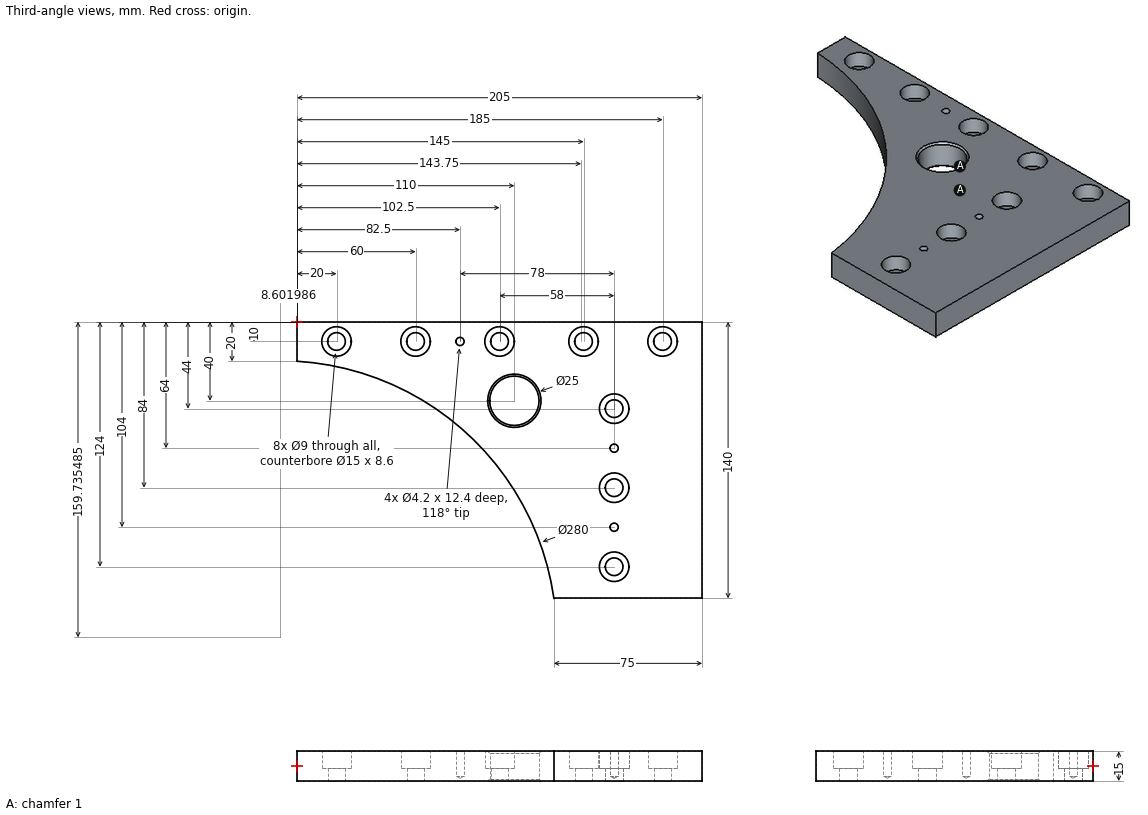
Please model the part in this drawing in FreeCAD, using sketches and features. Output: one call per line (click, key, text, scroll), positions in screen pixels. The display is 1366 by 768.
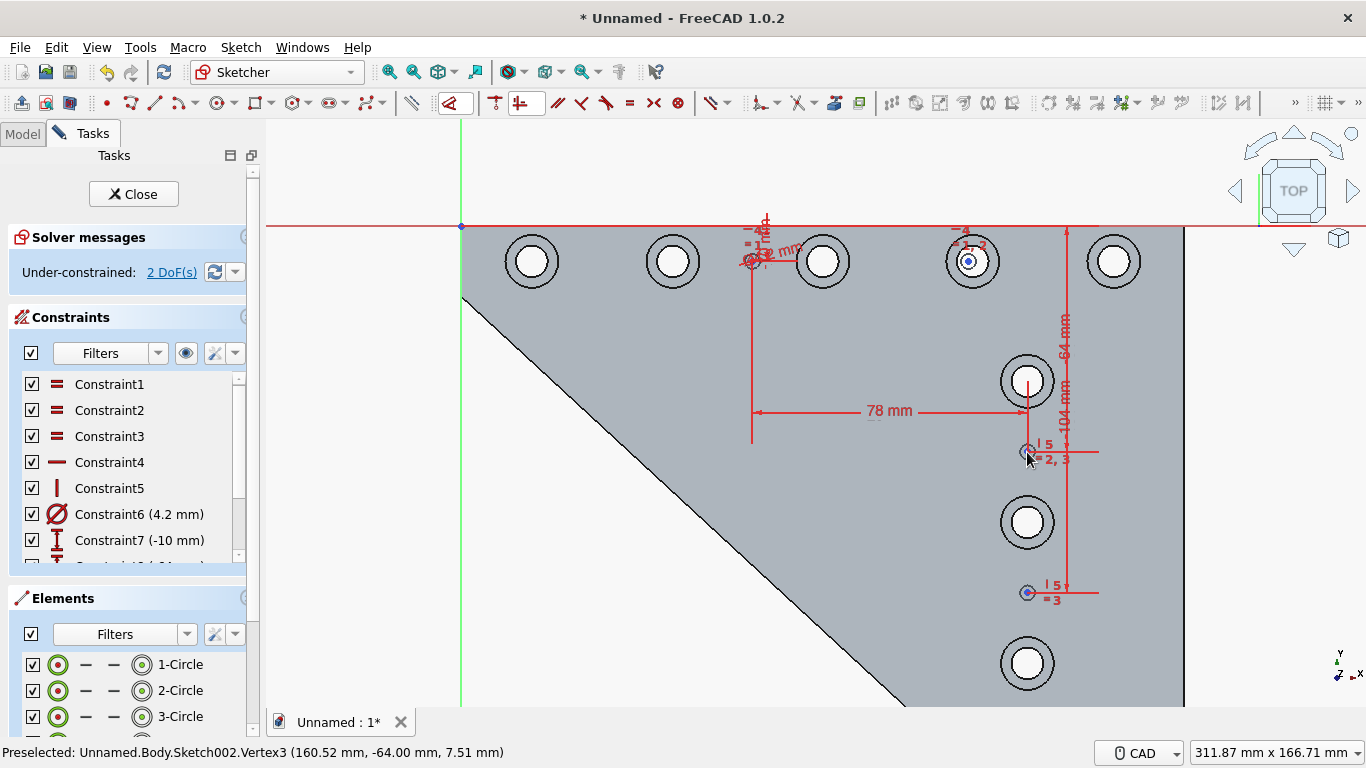
click(752, 261)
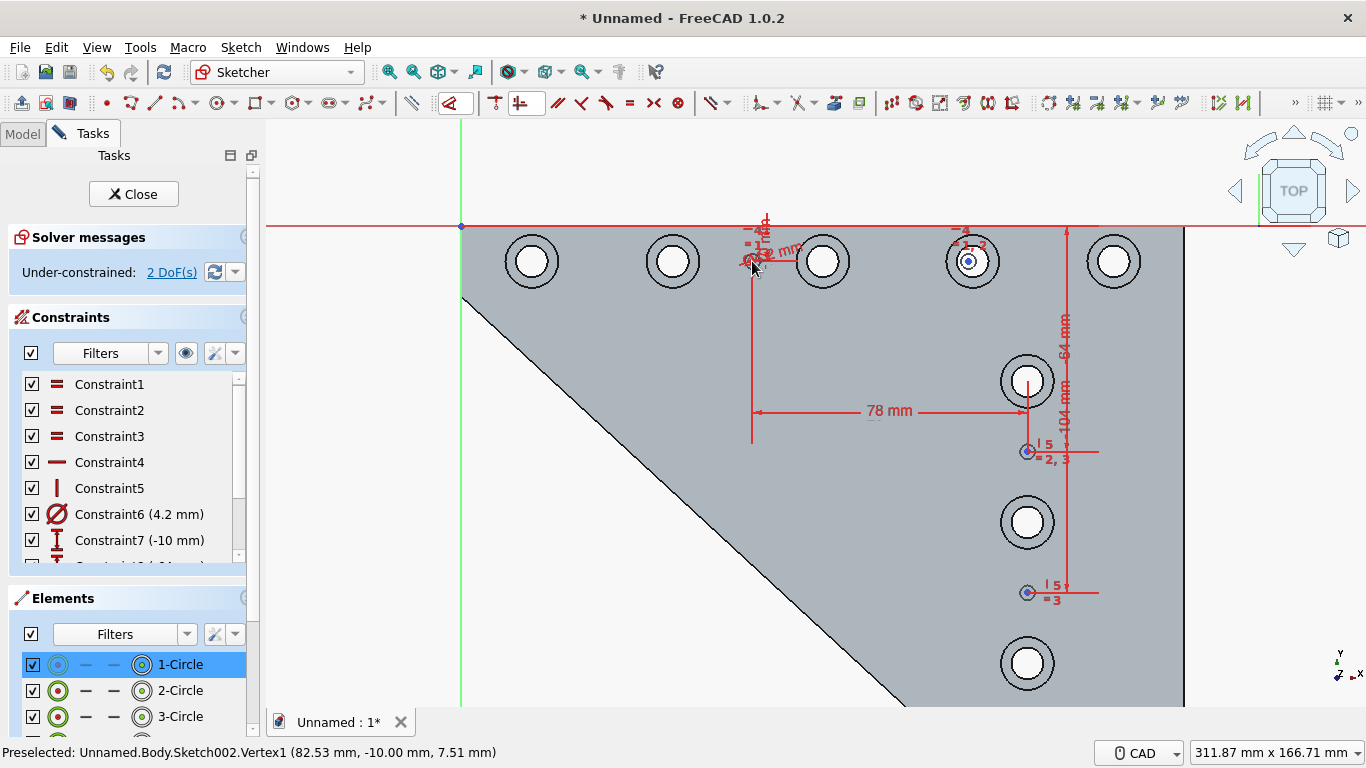
click(468, 104)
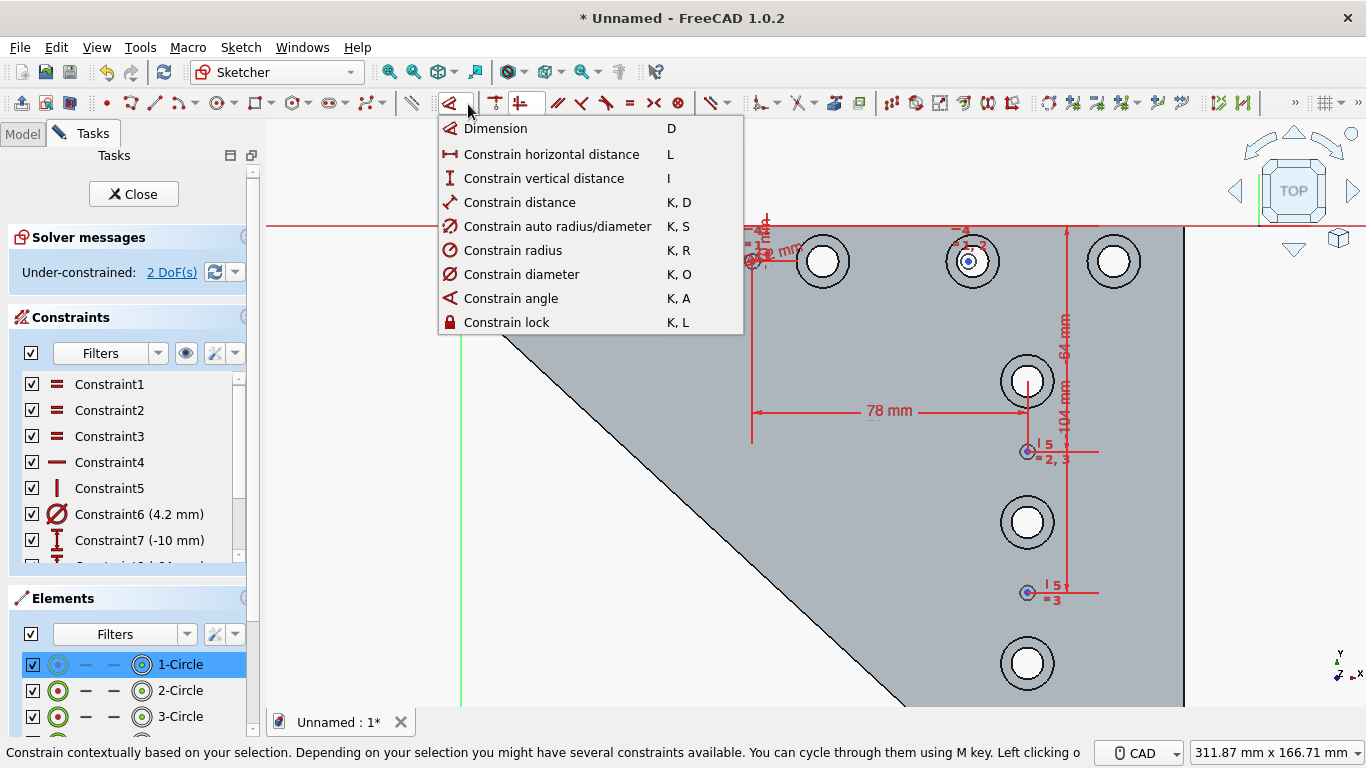
click(591, 154)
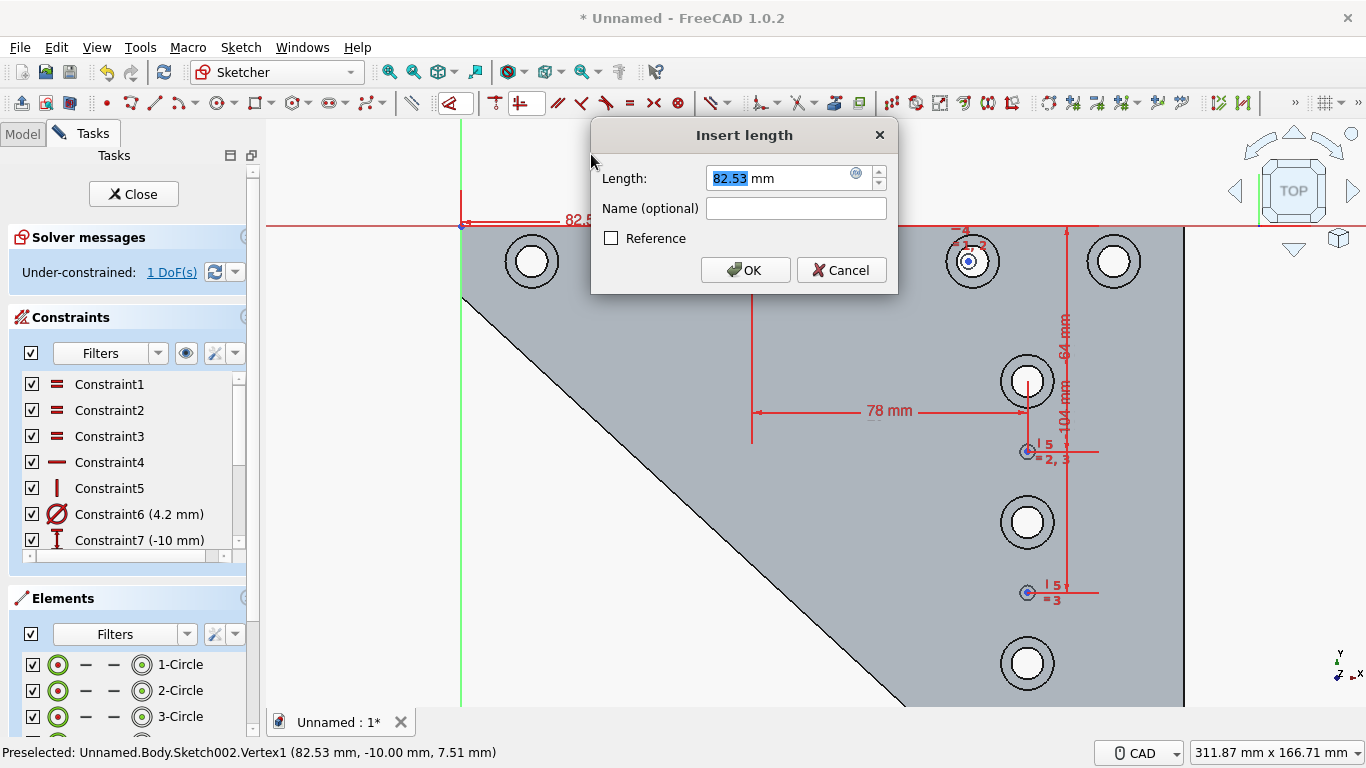
text(82.5)
key(Return)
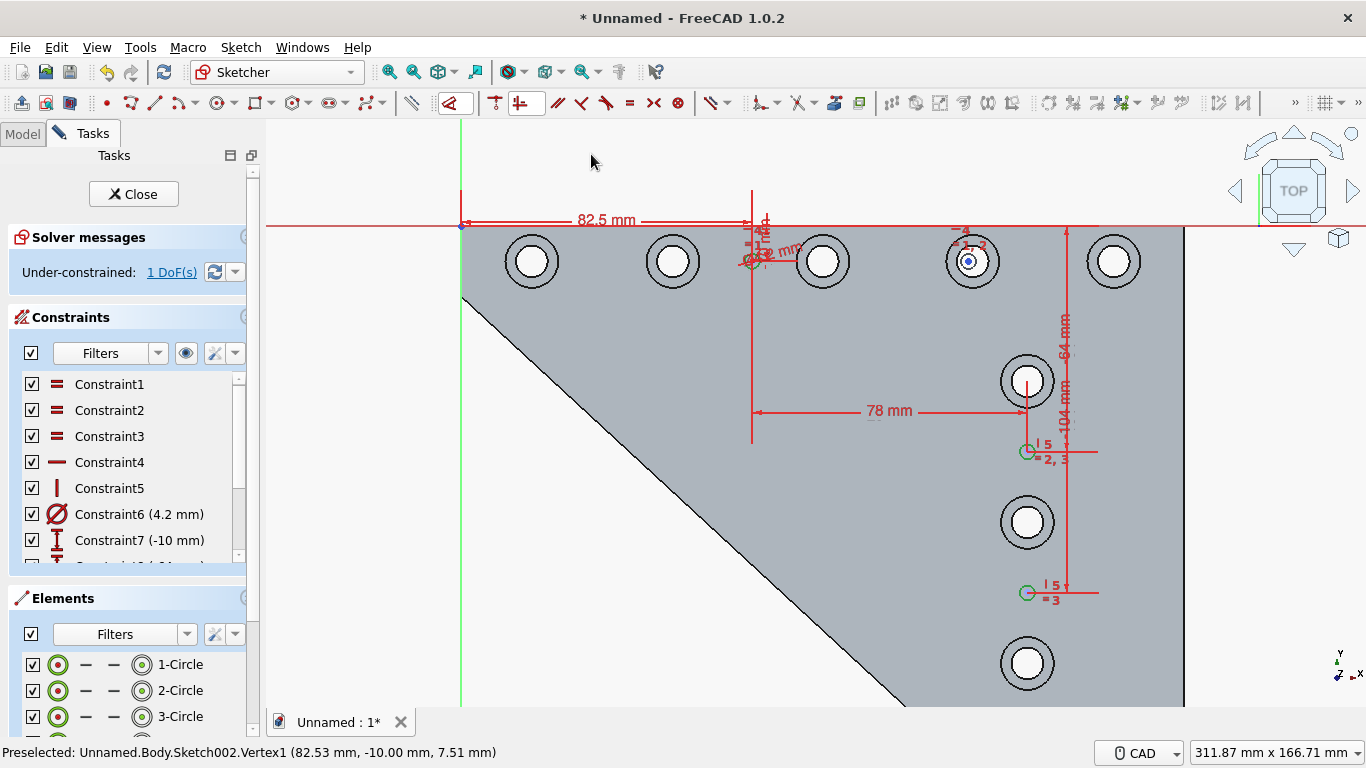
click(968, 261)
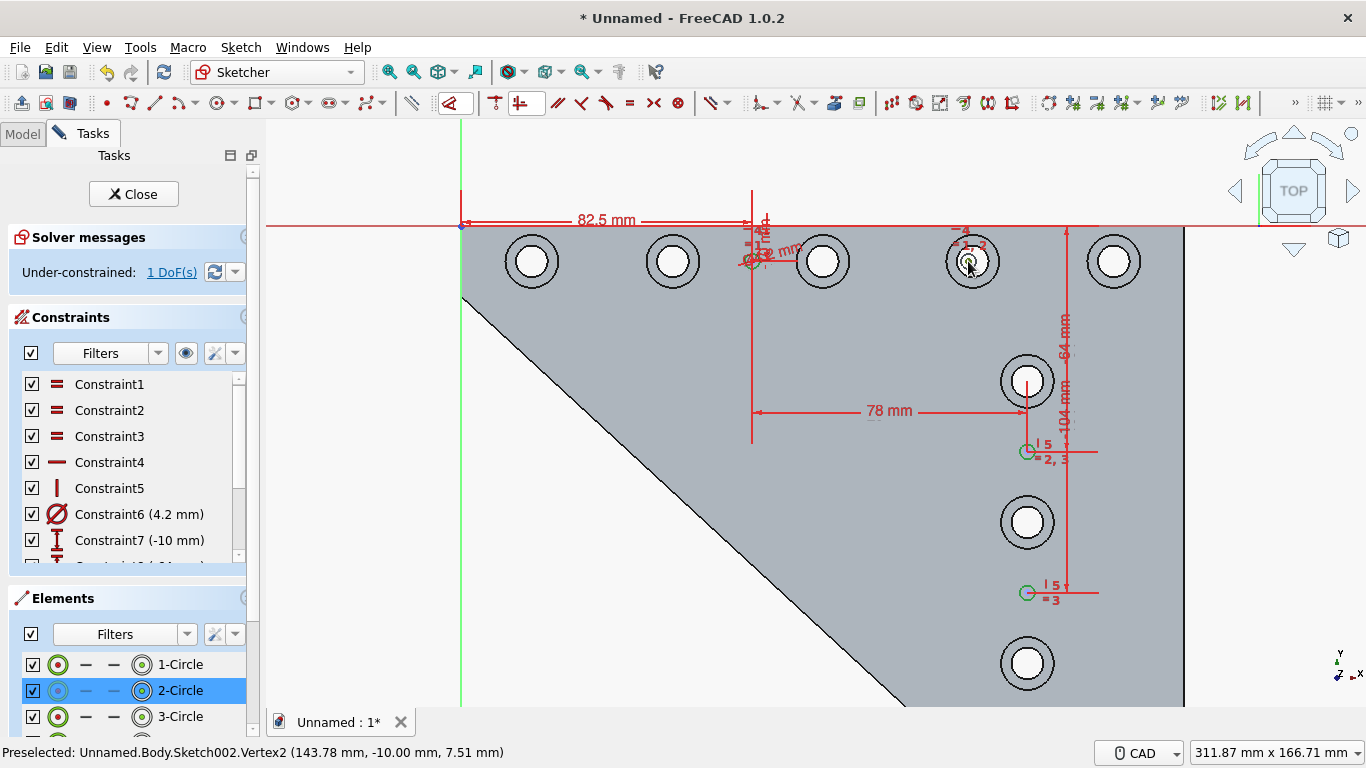
click(468, 104)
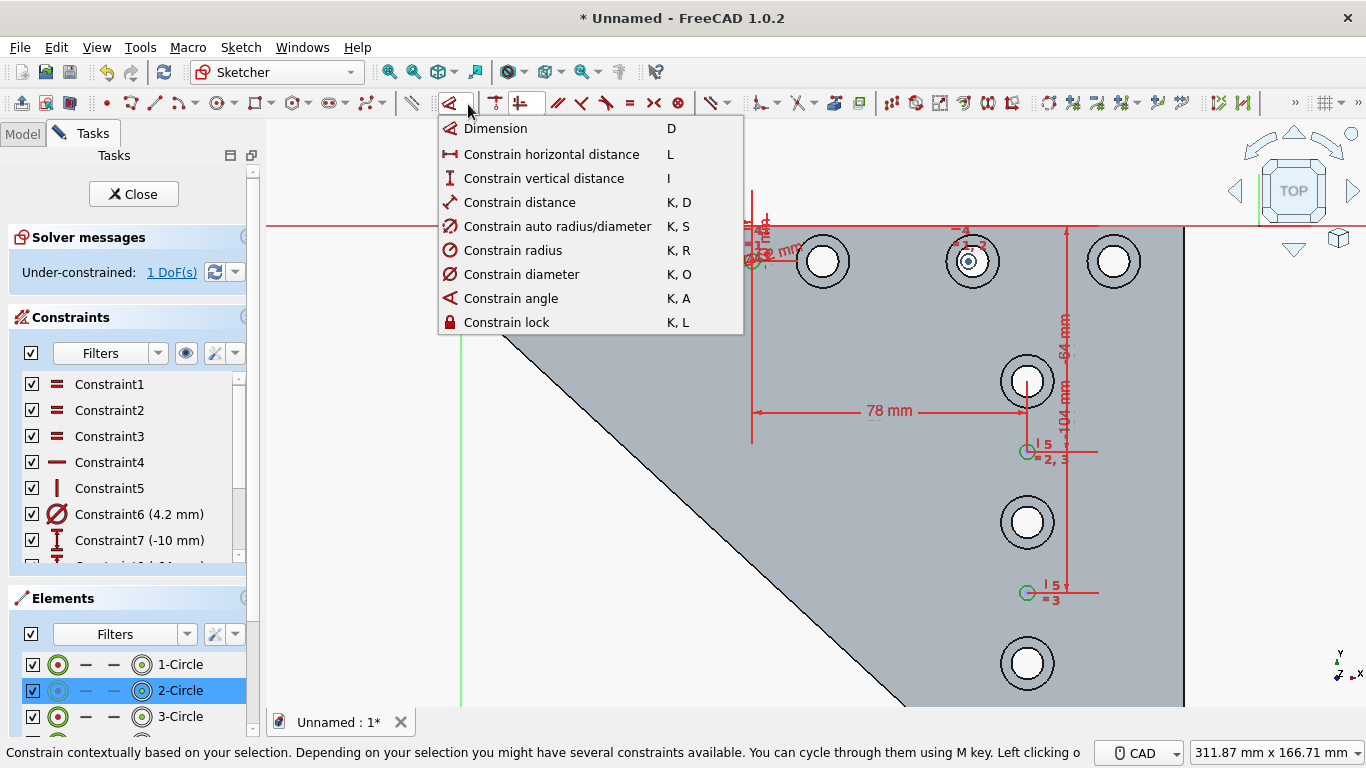
click(591, 154)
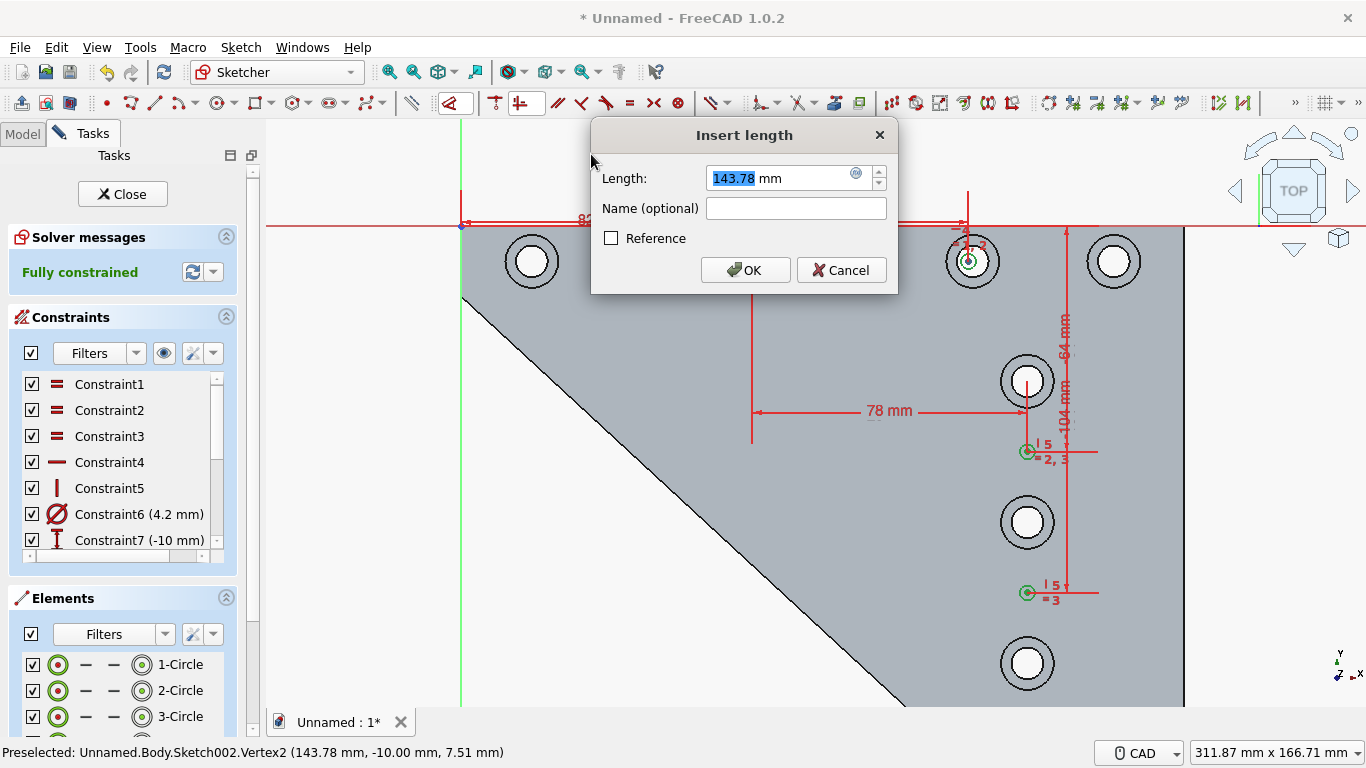
text(143.75)
key(Return)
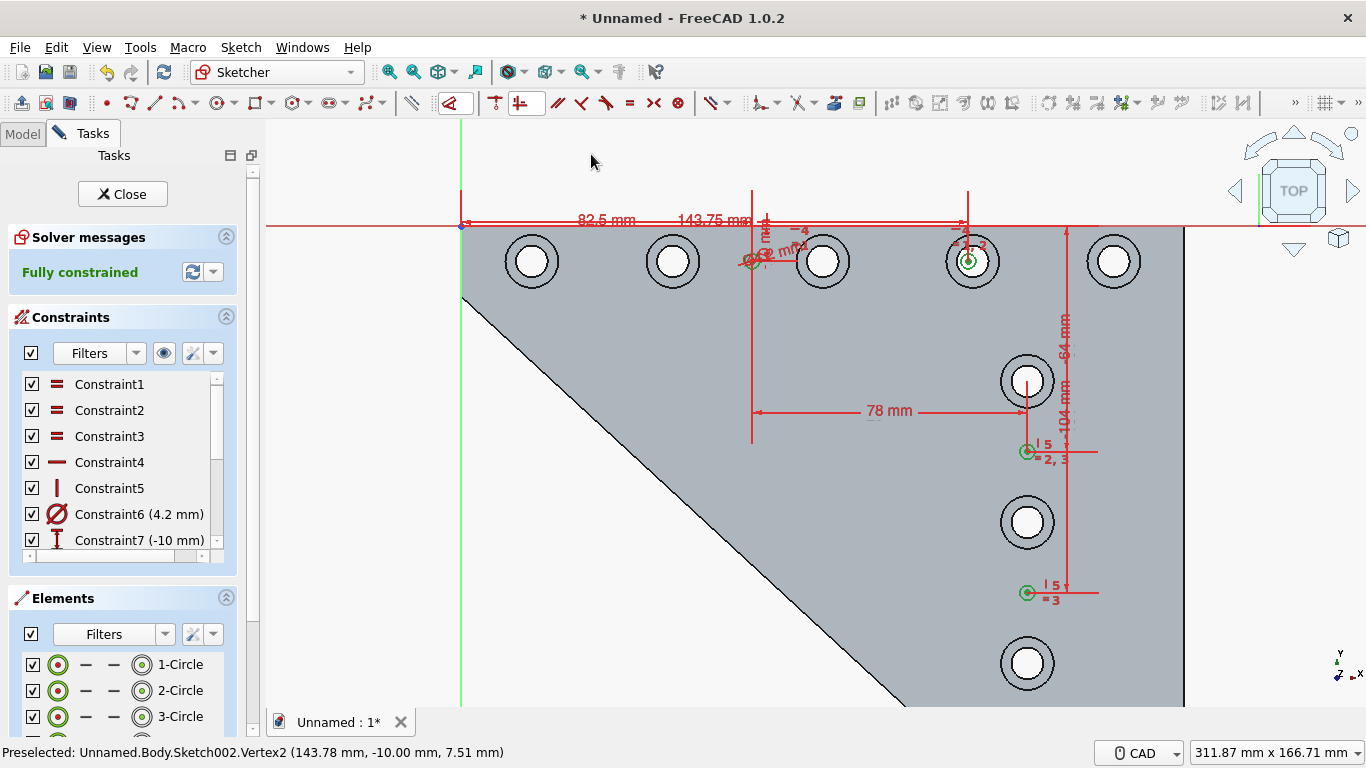
click(123, 194)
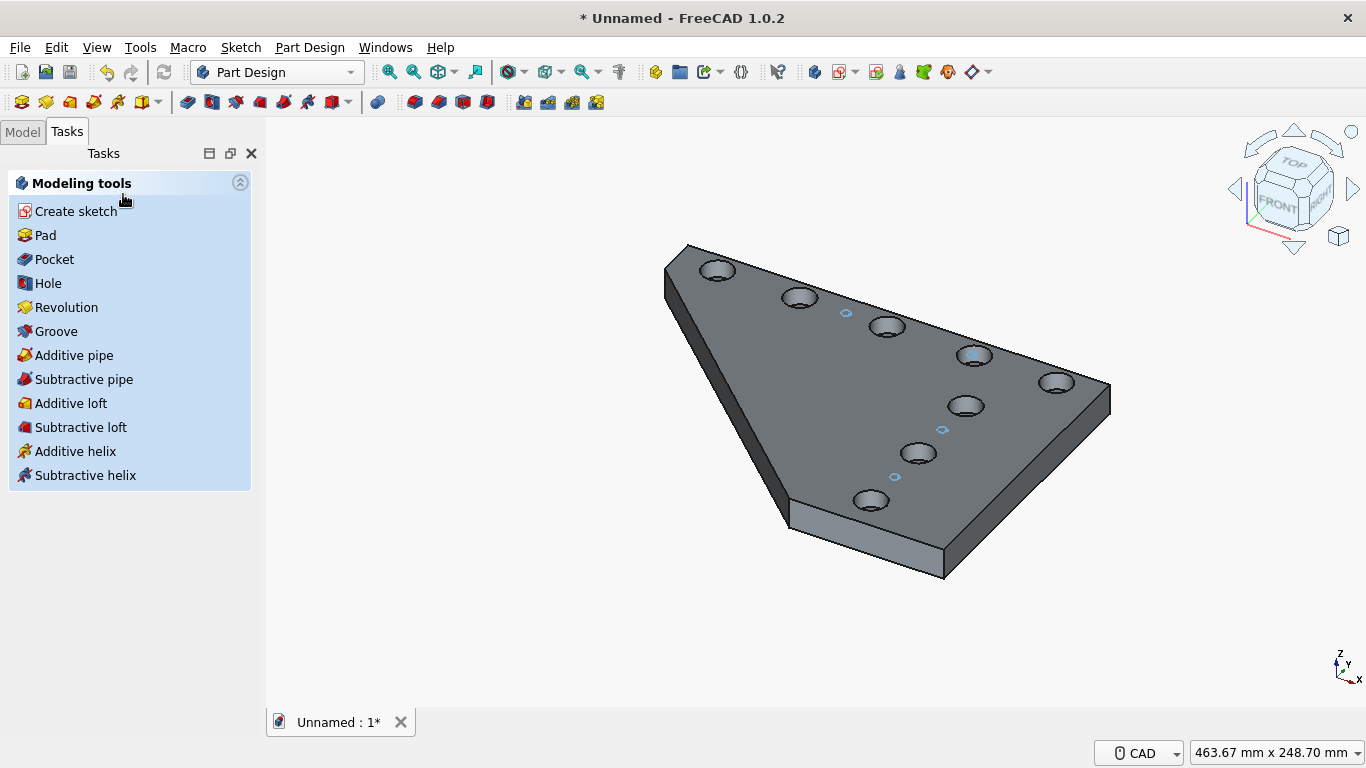
click(212, 102)